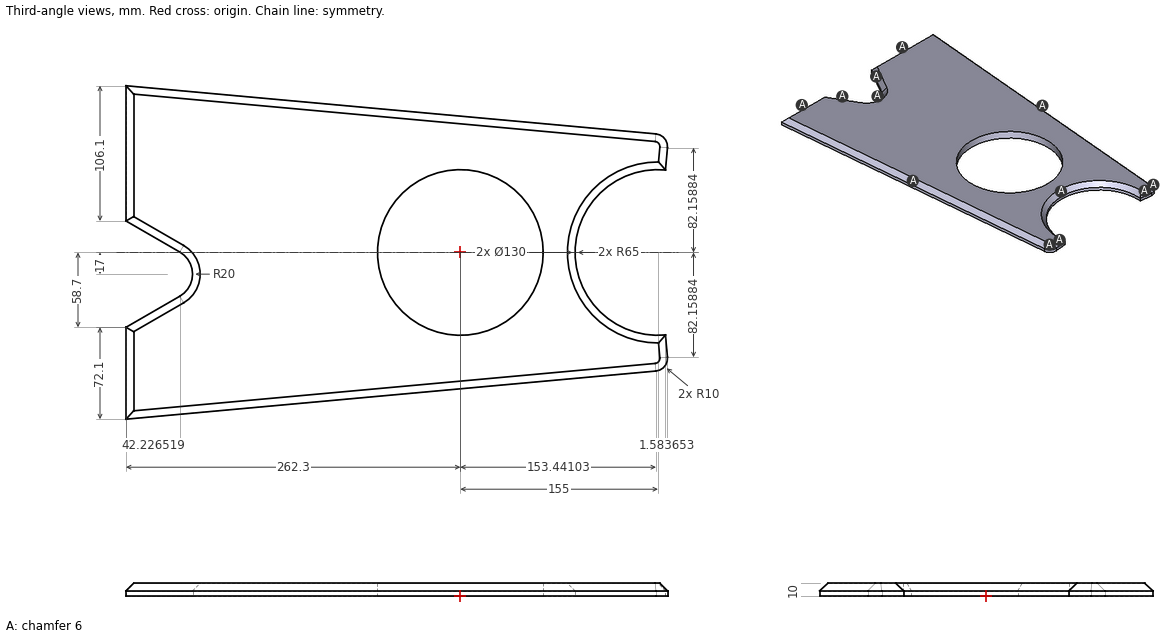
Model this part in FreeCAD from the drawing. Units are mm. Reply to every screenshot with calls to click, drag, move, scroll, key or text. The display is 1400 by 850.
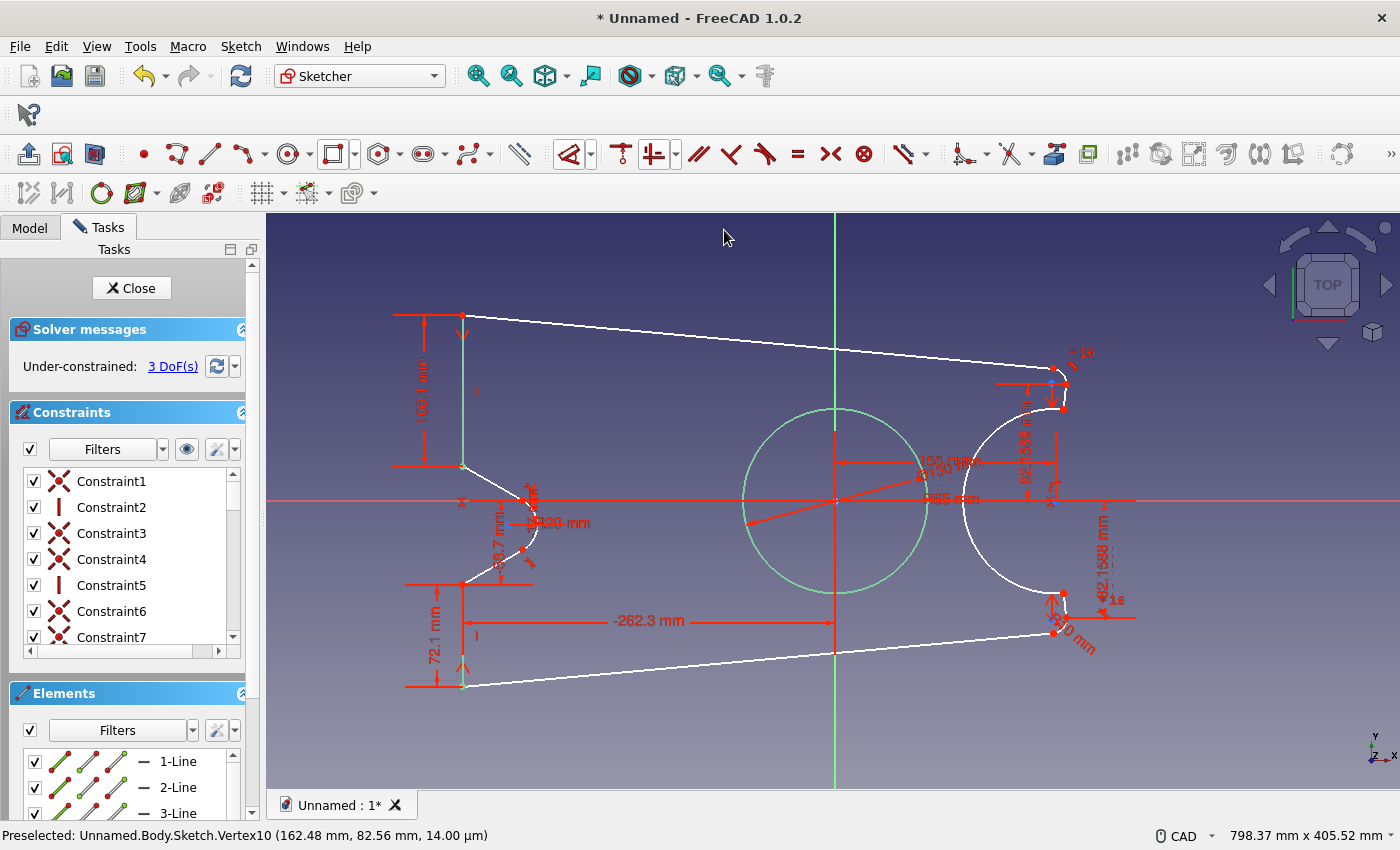
scroll(1065, 608, up, 15)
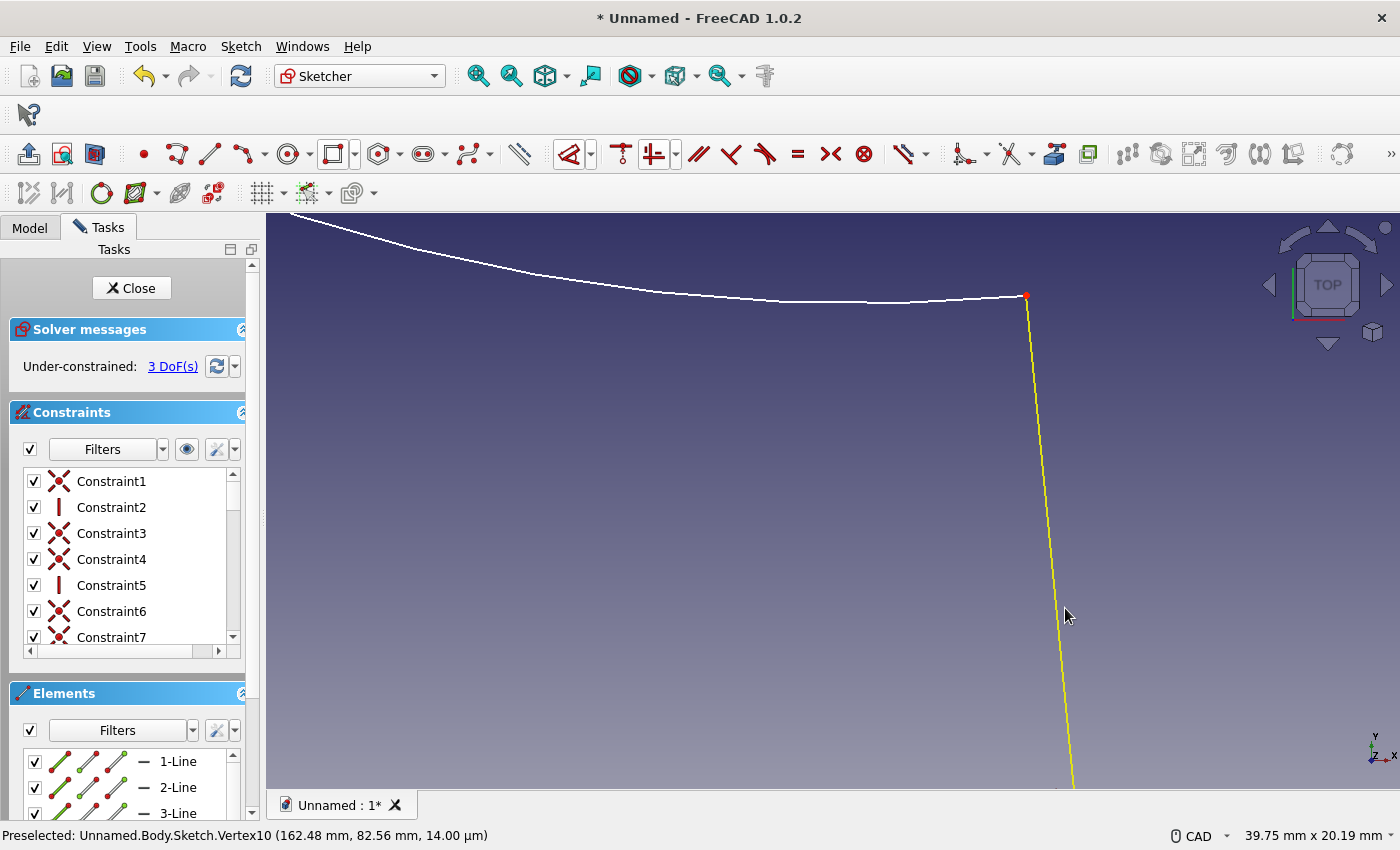
click(1055, 594)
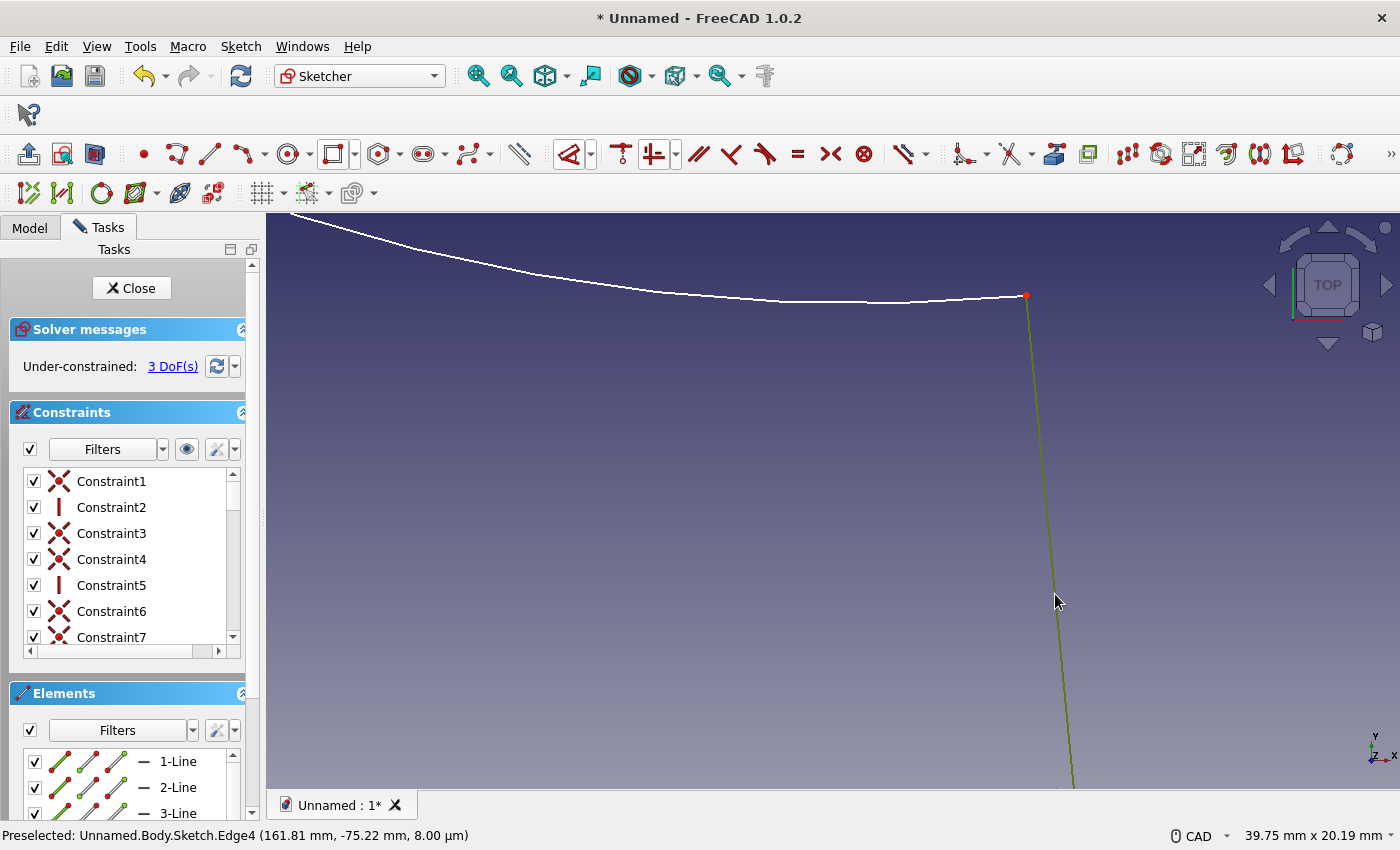
key(l)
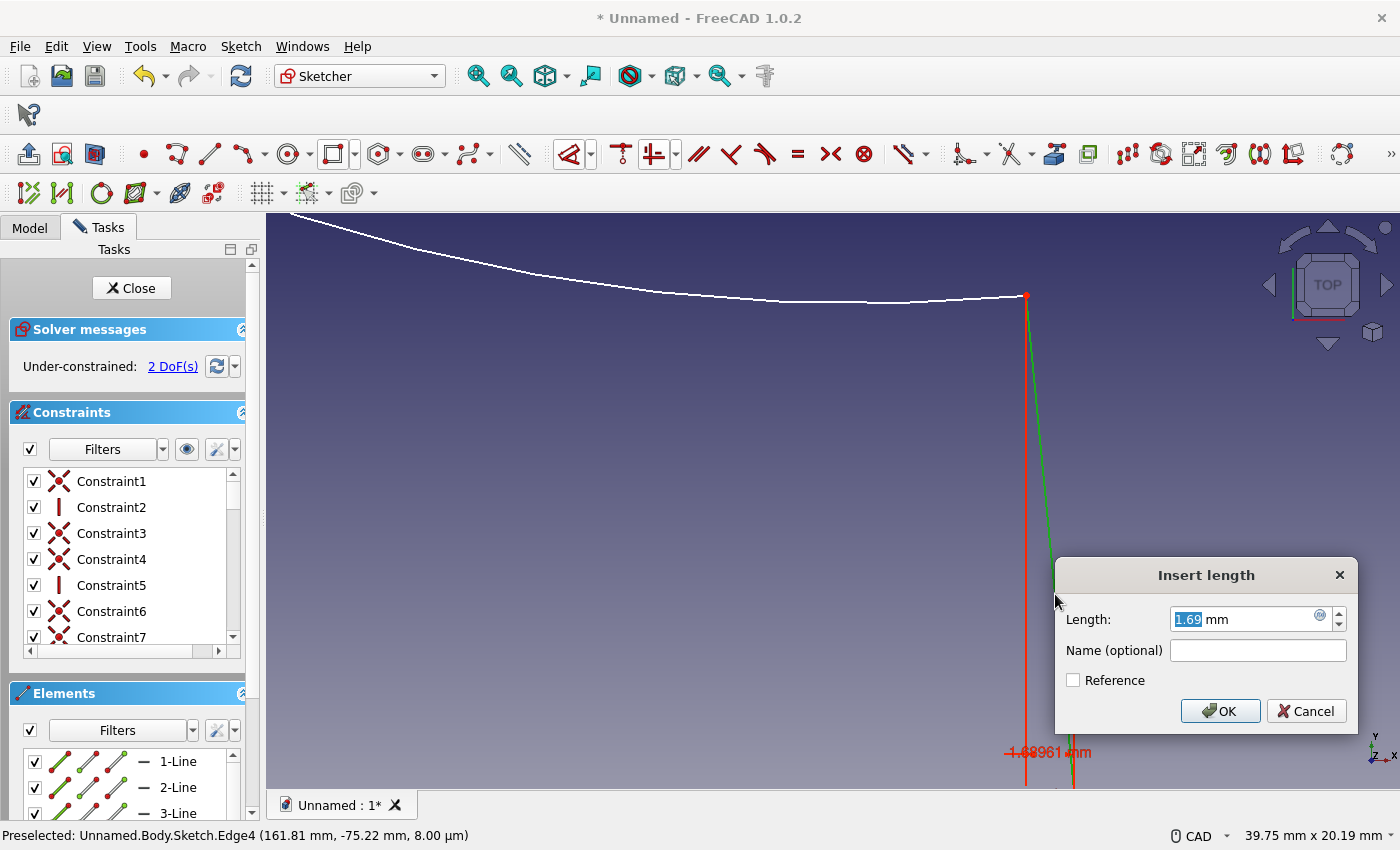
text(1.583653)
key(Return)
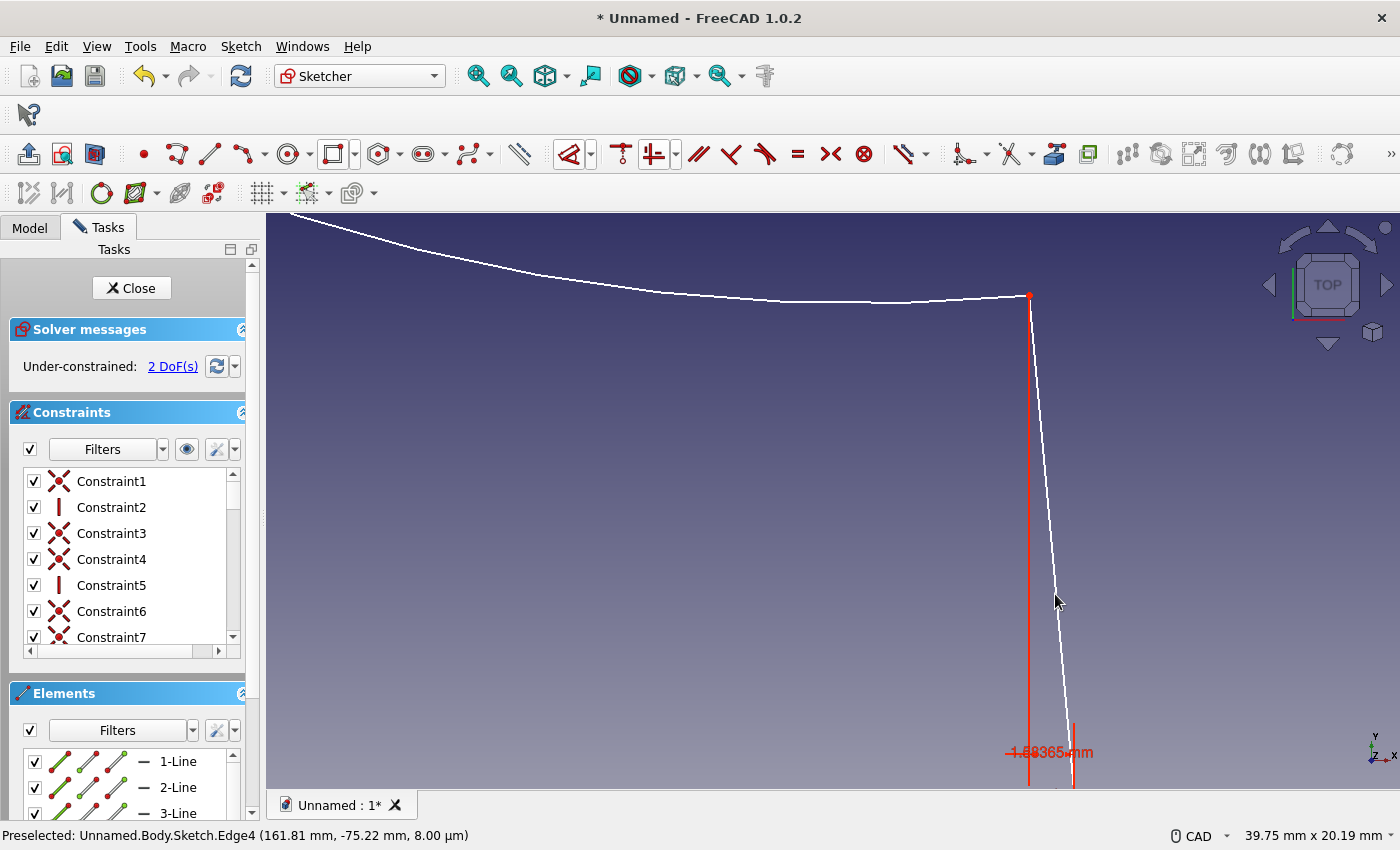
scroll(1066, 609, down, 15)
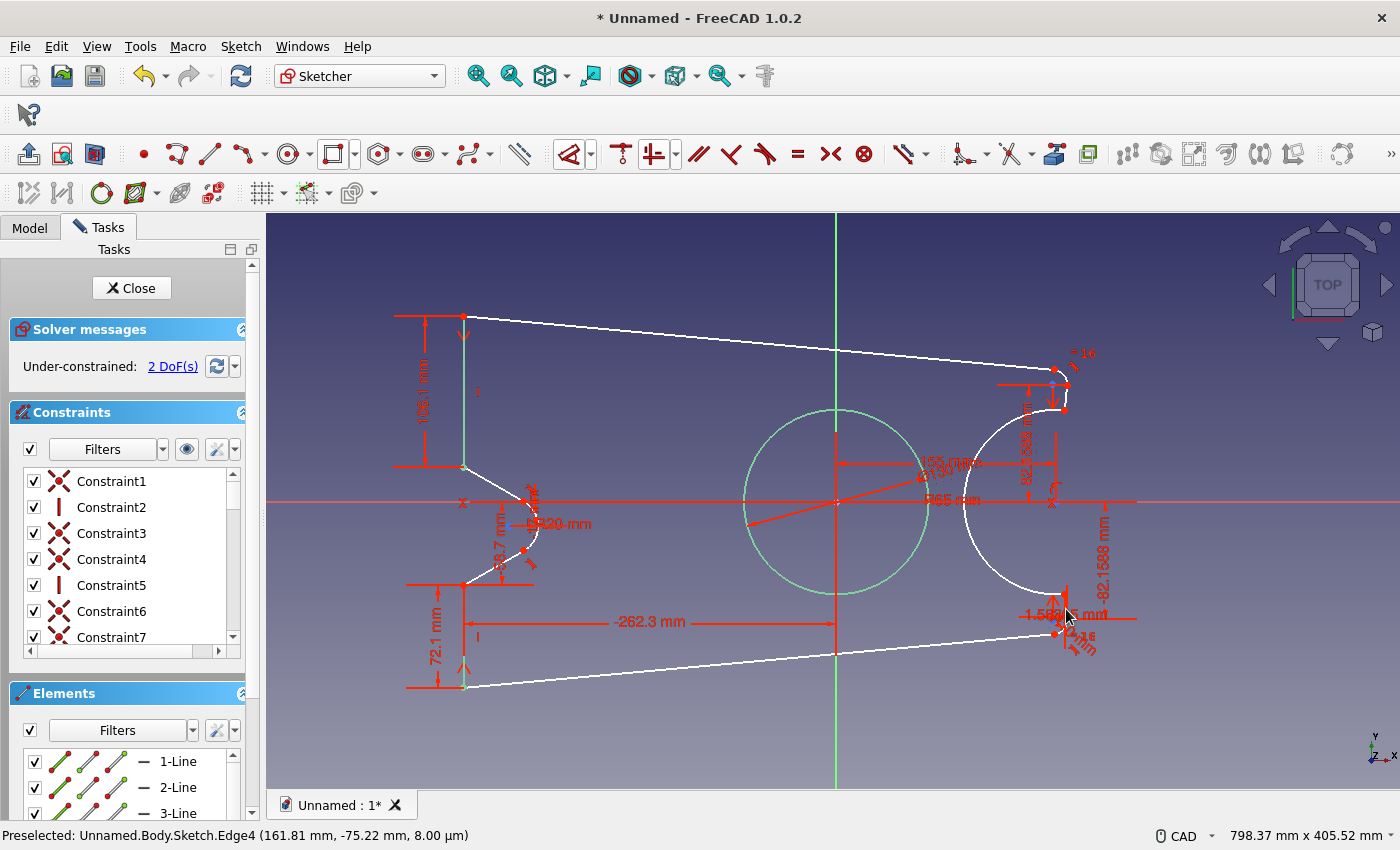
click(1054, 634)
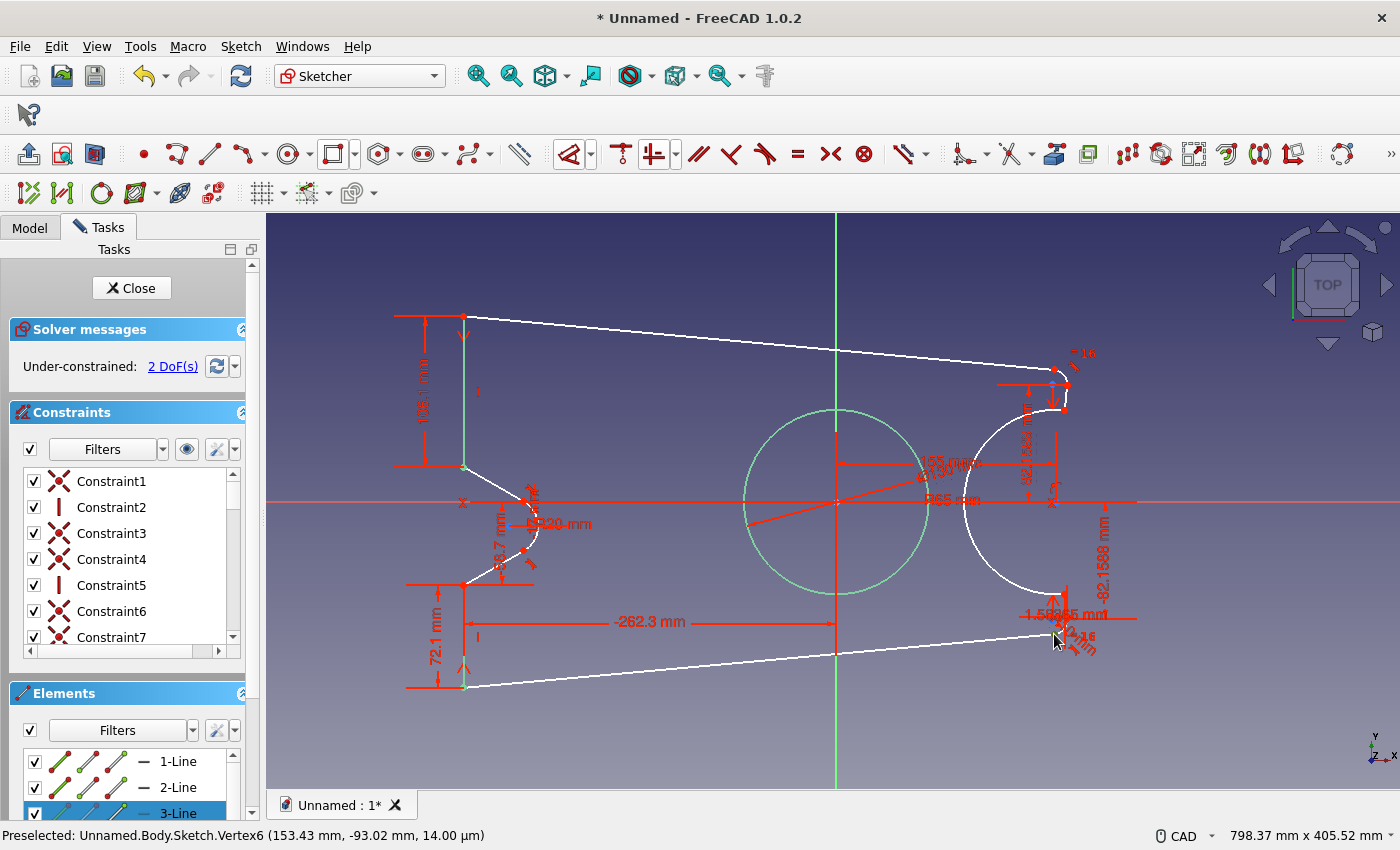
key(l)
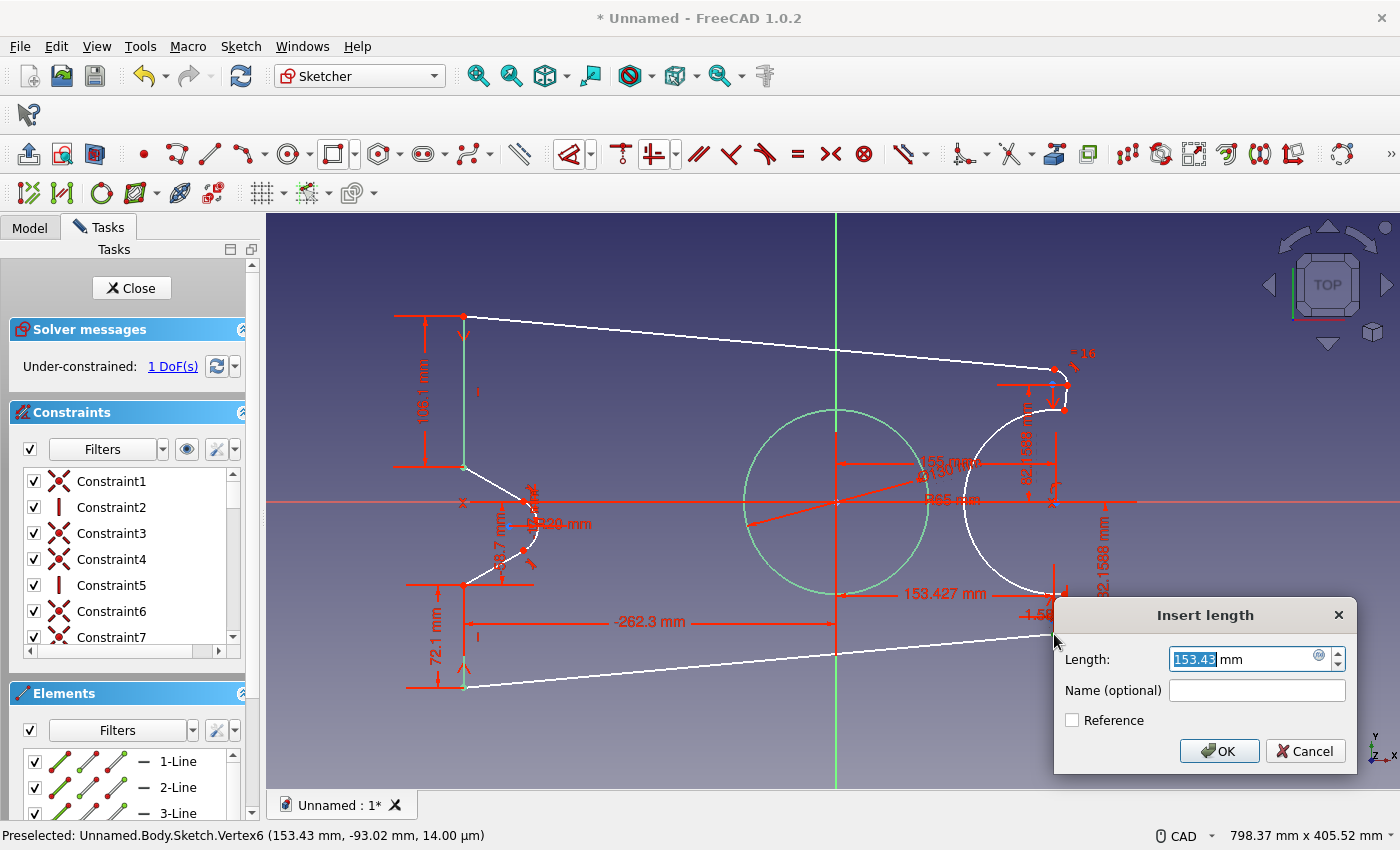
text(153.44103)
key(Return)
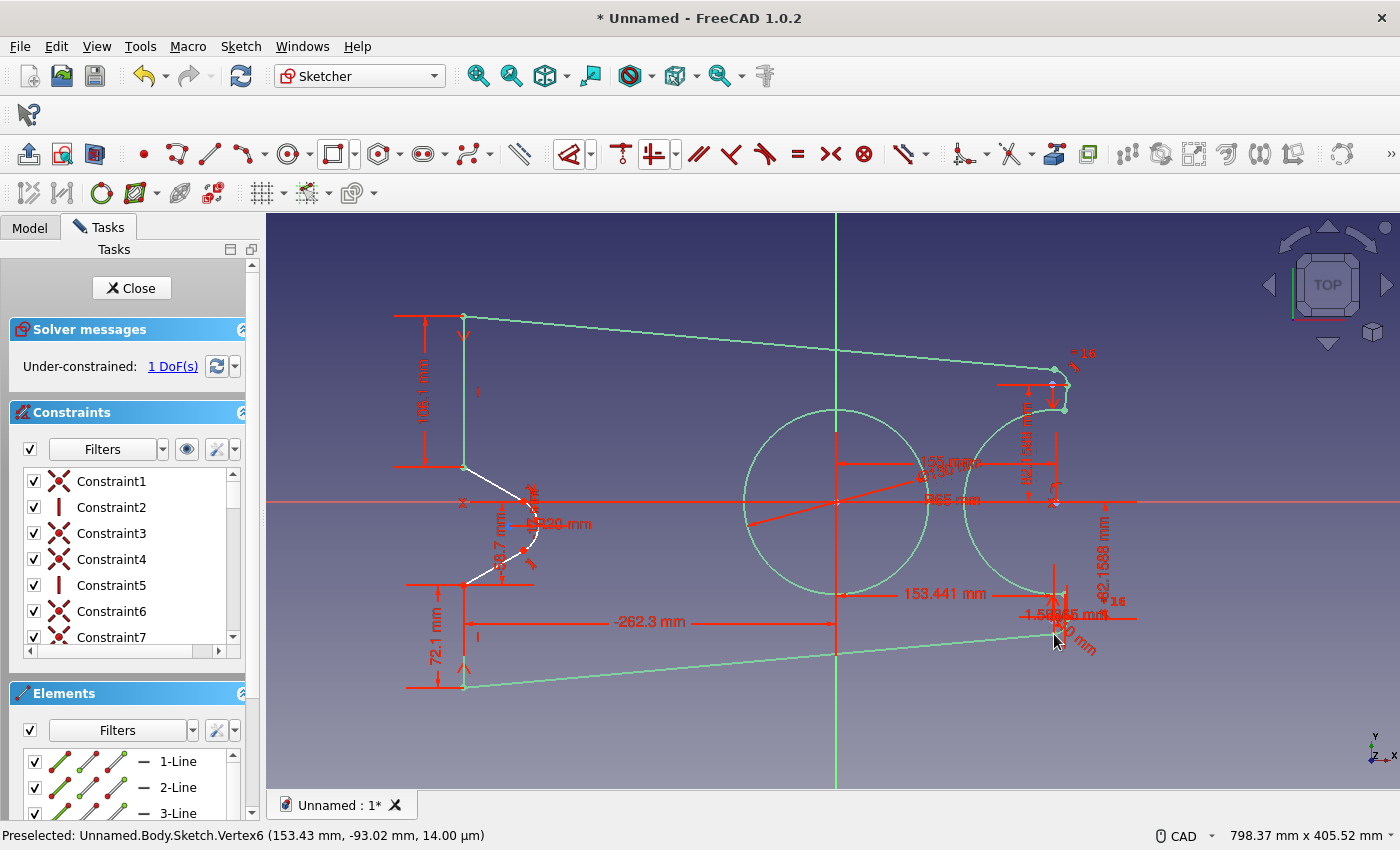
click(482, 575)